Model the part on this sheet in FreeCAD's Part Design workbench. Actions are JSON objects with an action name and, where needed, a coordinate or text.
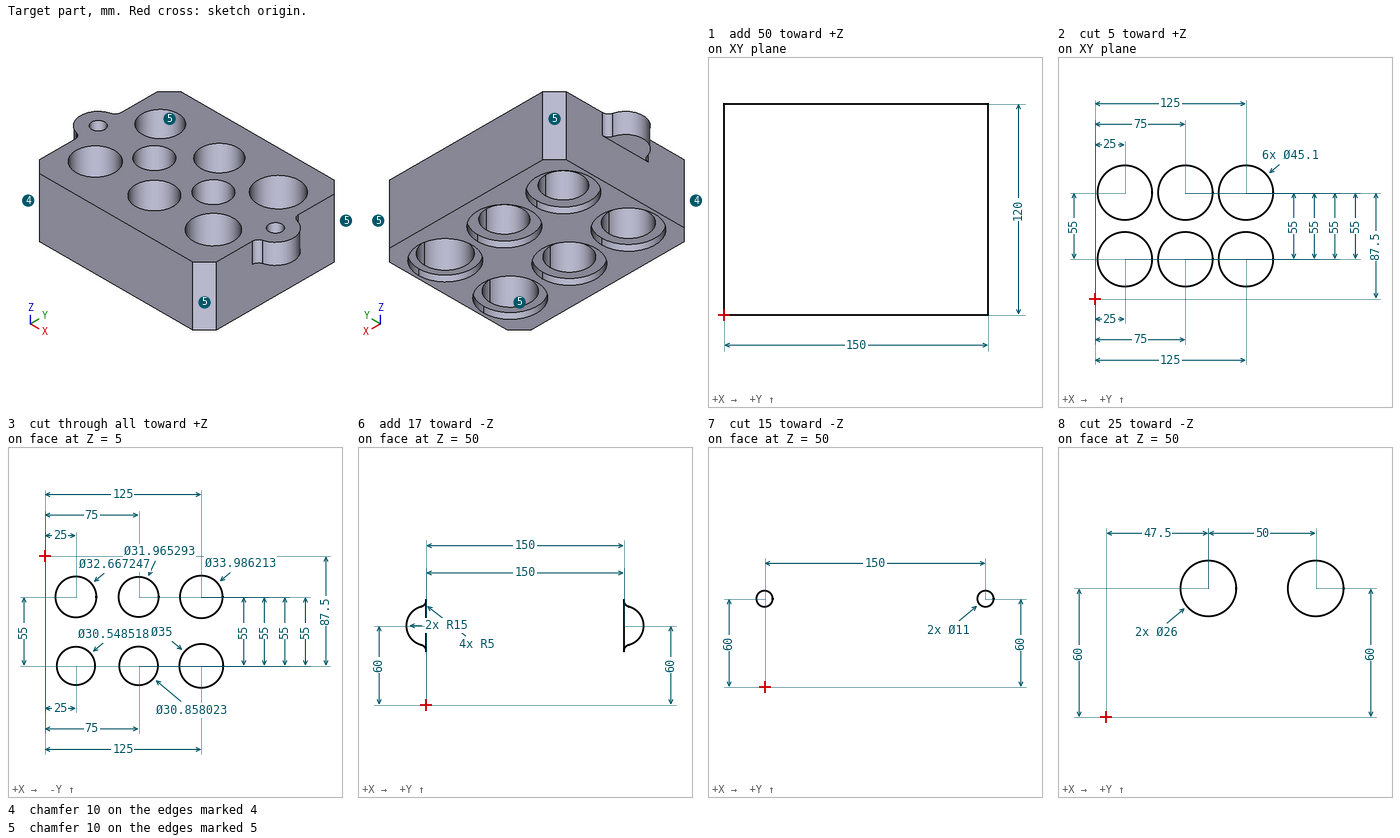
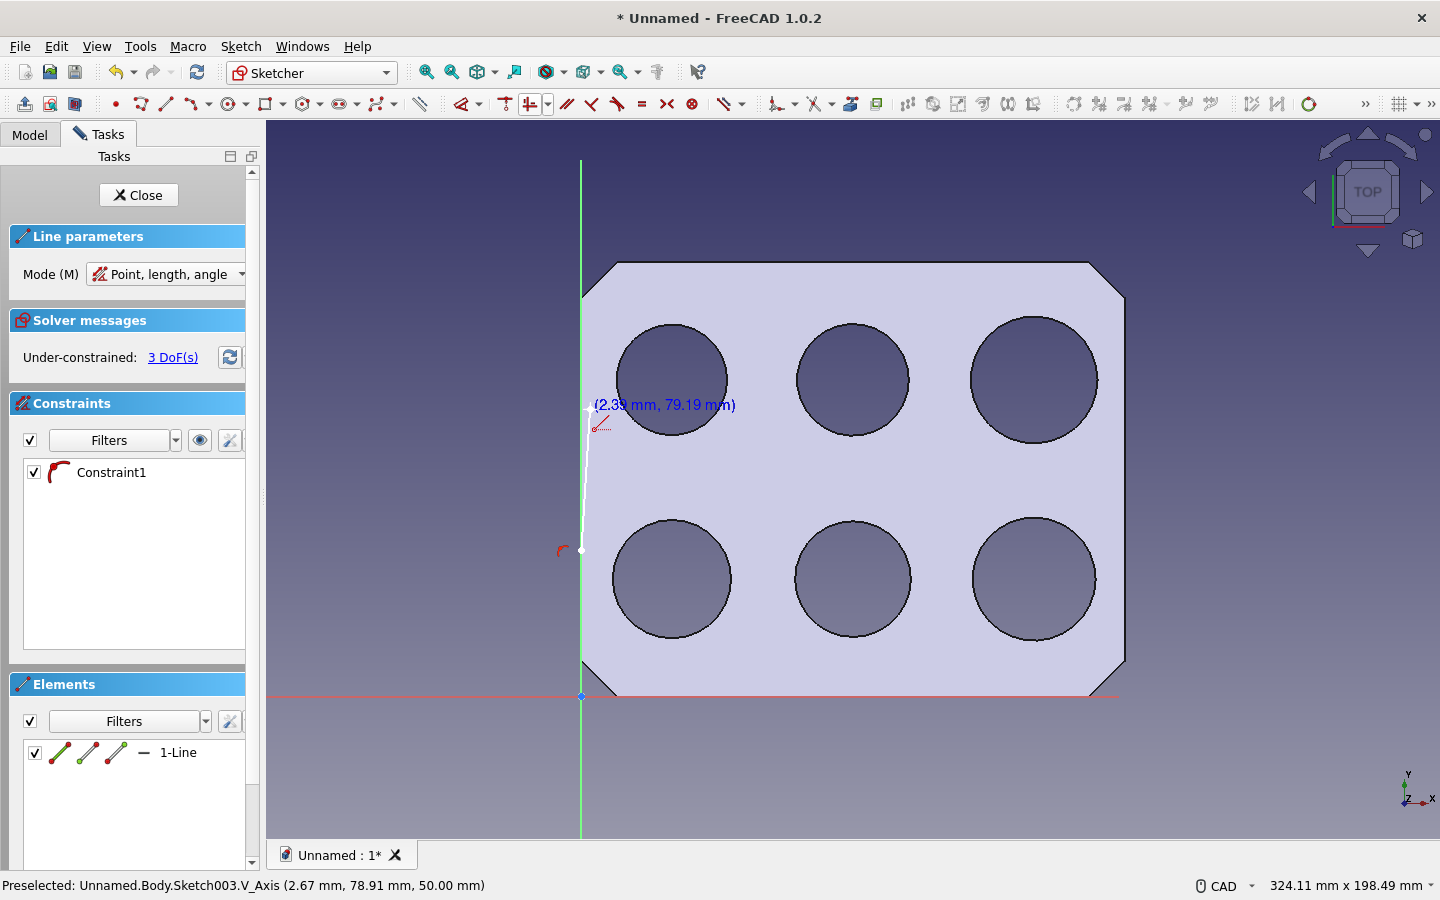
{"action": "key", "text": "g 3 a"}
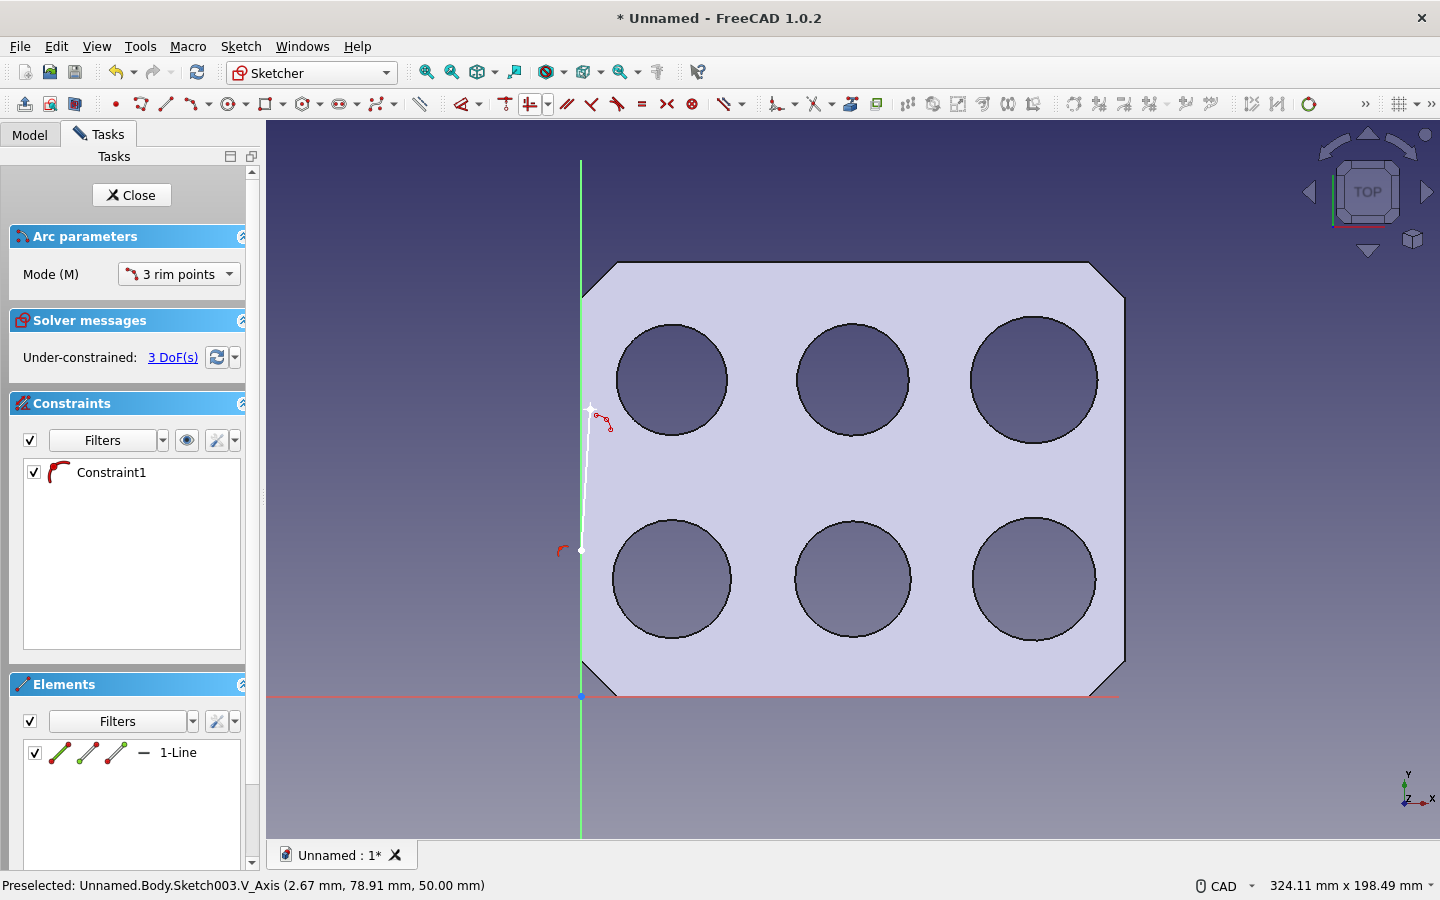
{"action": "left_click", "coordinate": [590, 410]}
{"action": "left_click", "coordinate": [568, 427]}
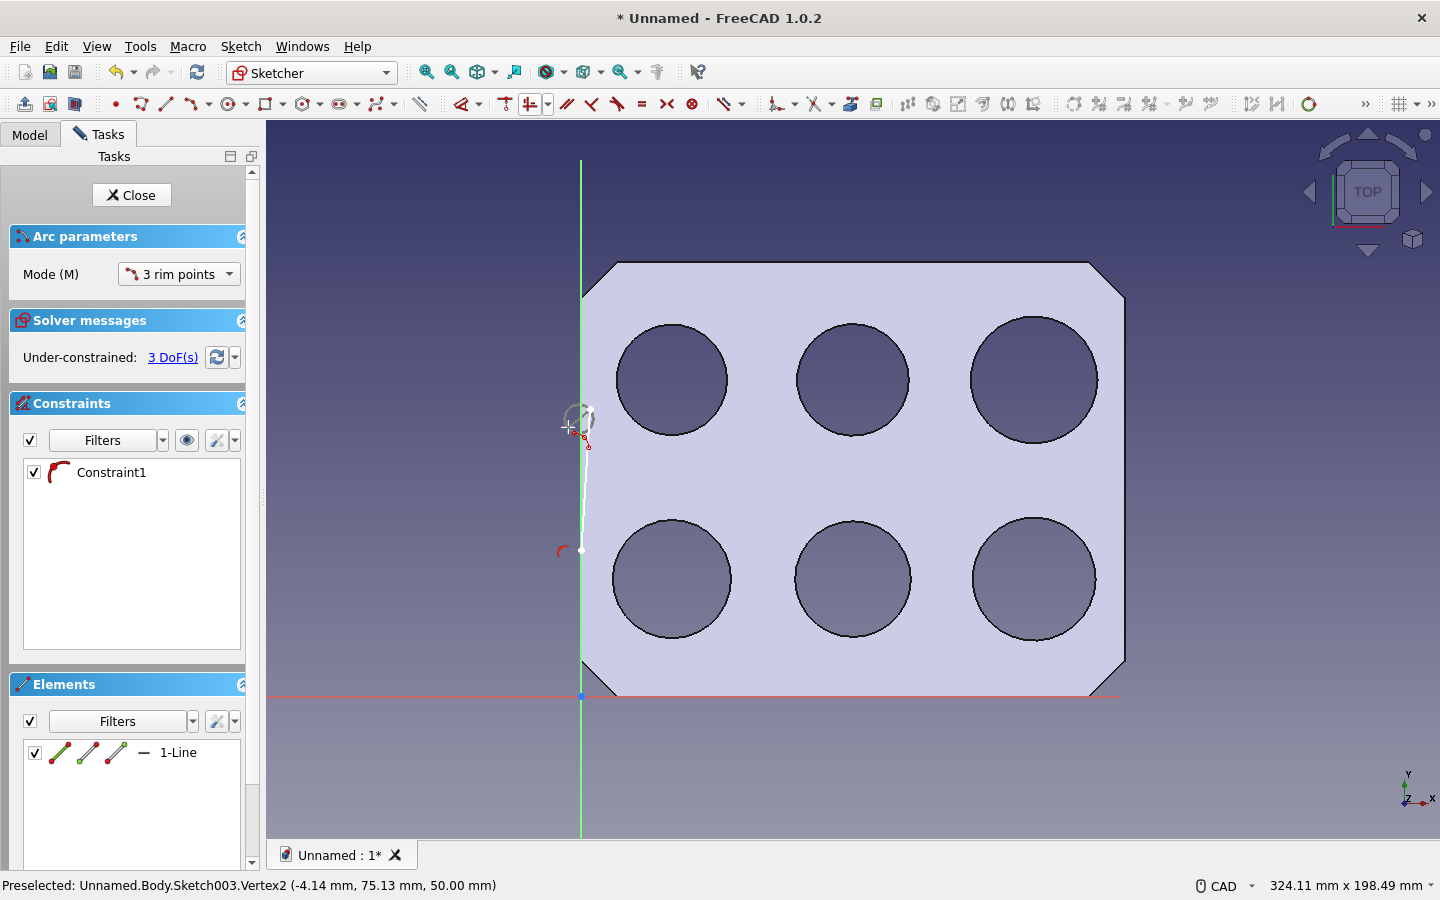
{"action": "scroll", "coordinate": [578, 420], "scroll_direction": "up", "scroll_amount": 8}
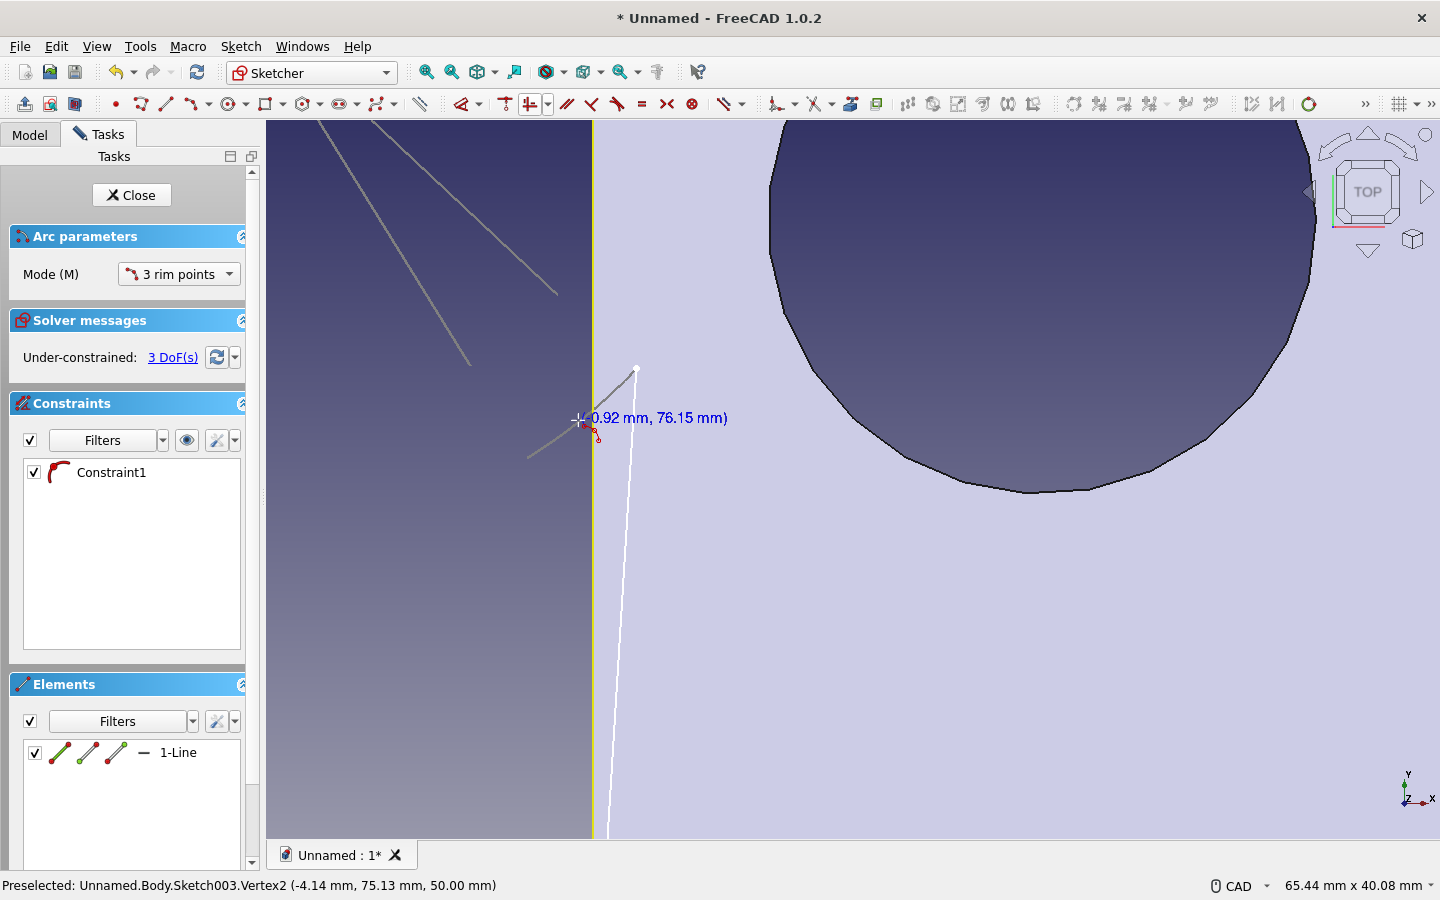
{"action": "left_click", "coordinate": [575, 421]}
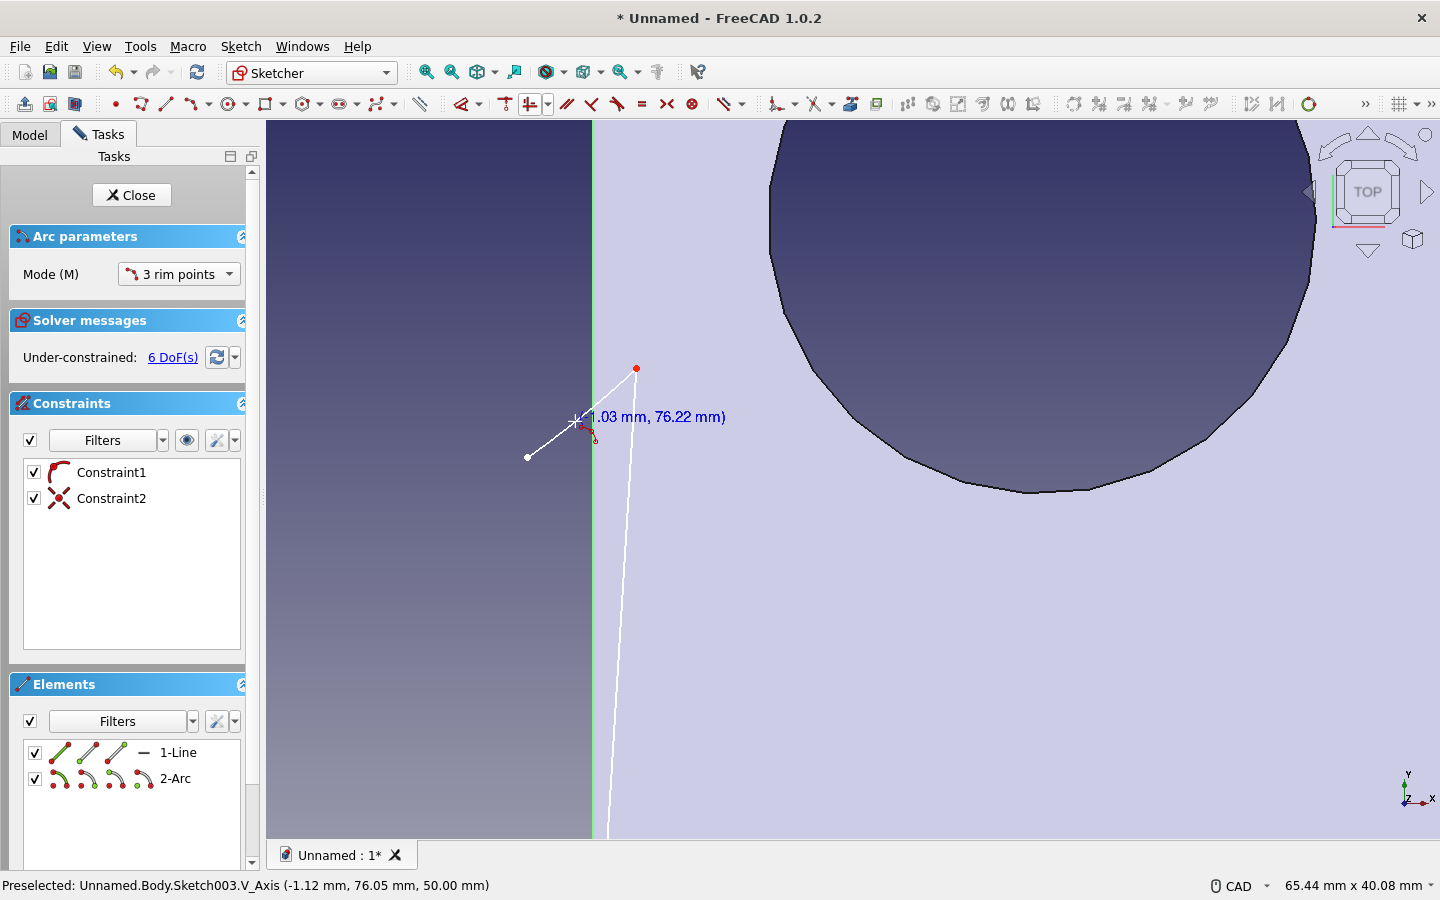
{"action": "scroll", "coordinate": [492, 328], "scroll_direction": "down", "scroll_amount": 8}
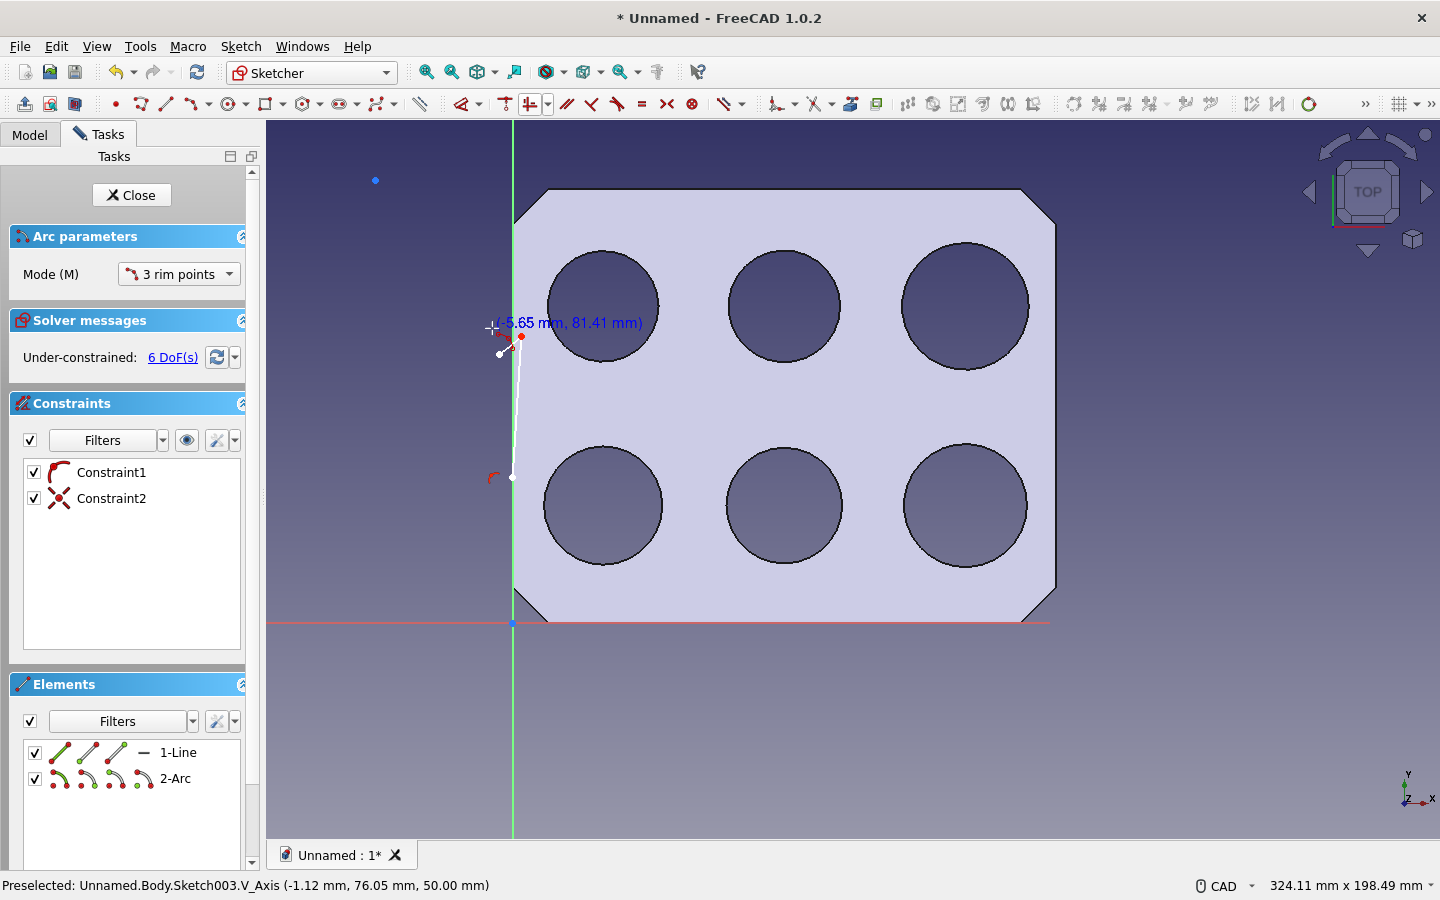
{"action": "left_click", "coordinate": [499, 354]}
{"action": "left_click", "coordinate": [499, 459]}
{"action": "left_click", "coordinate": [458, 406]}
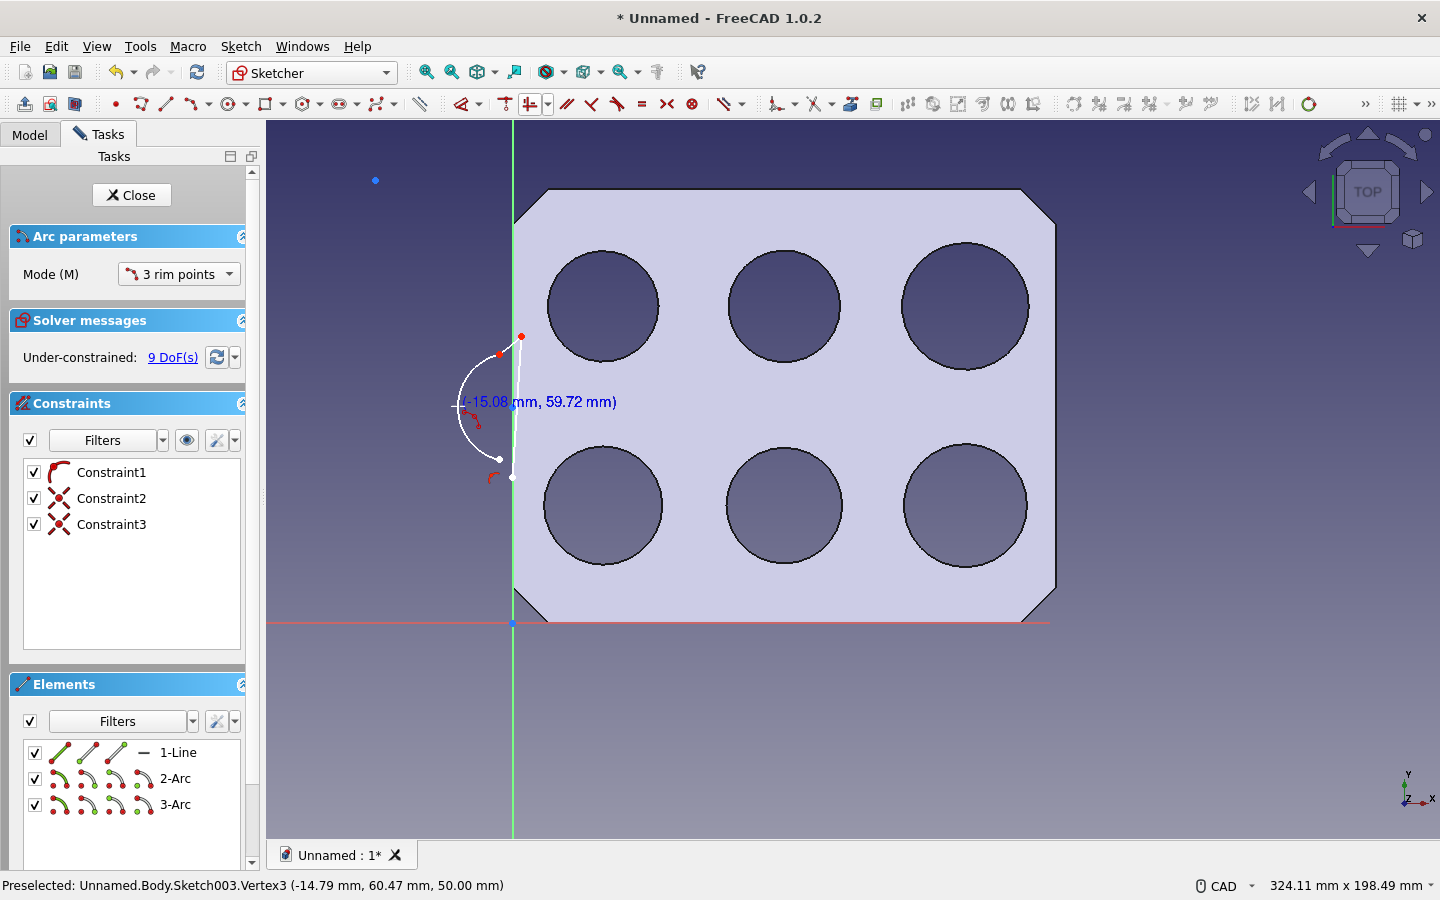
{"action": "left_click", "coordinate": [499, 460]}
{"action": "left_click", "coordinate": [513, 477]}